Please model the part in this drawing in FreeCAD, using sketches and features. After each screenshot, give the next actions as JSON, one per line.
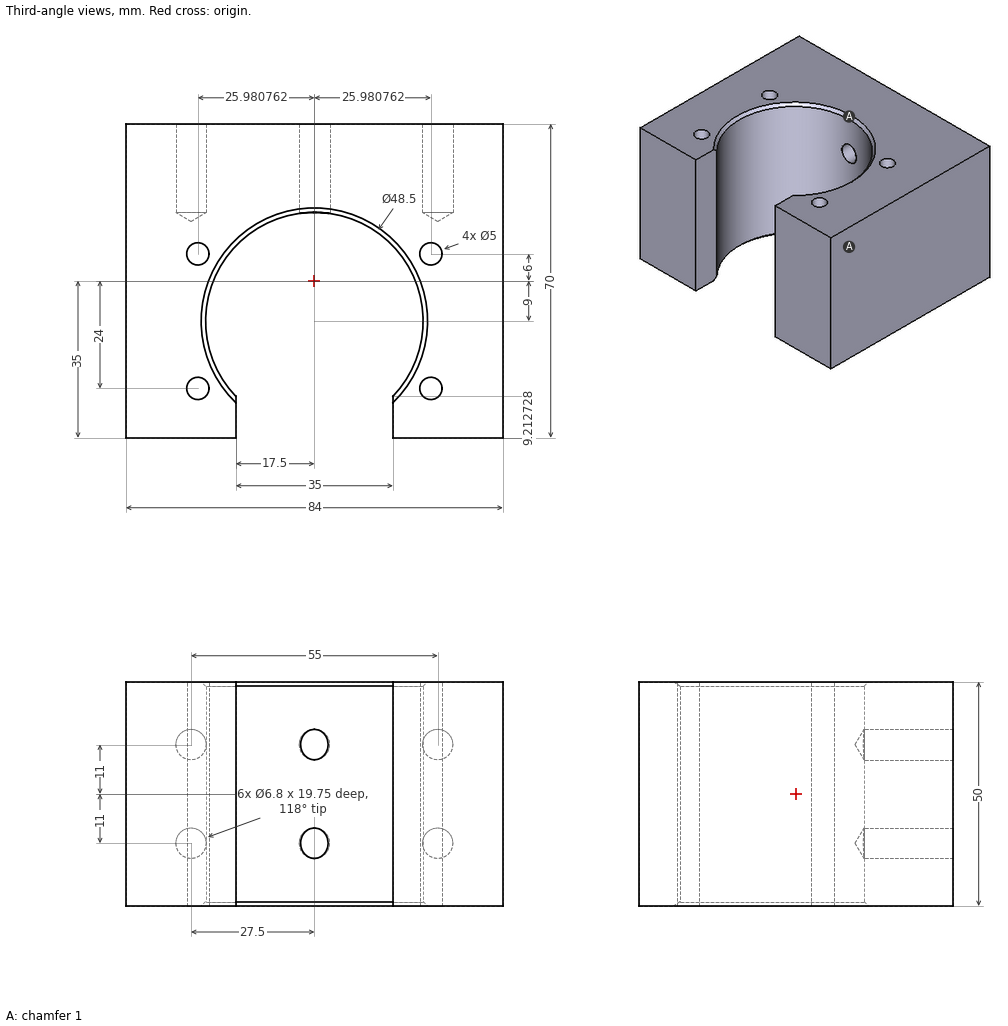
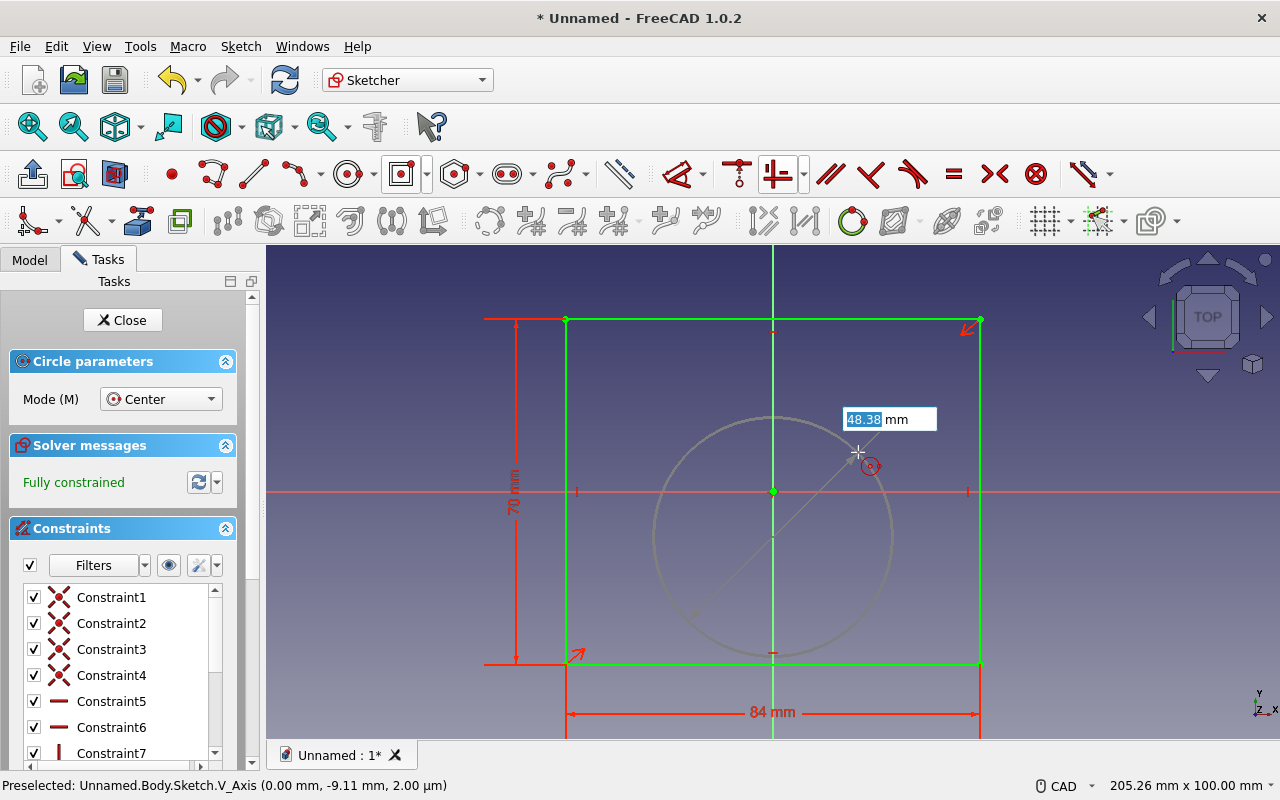
{"action": "type", "text": "48.5"}
{"action": "key", "text": "Return"}
{"action": "key", "text": "Escape"}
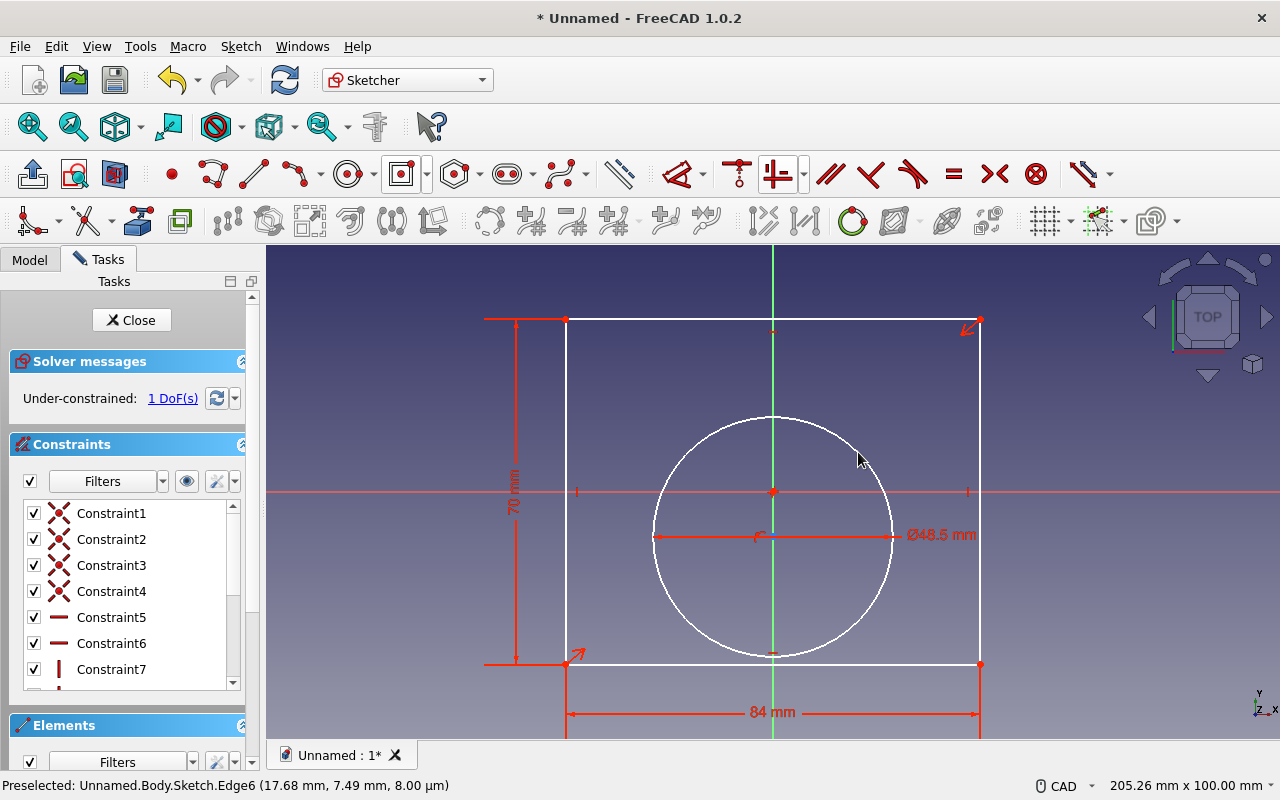
{"action": "key", "text": "d"}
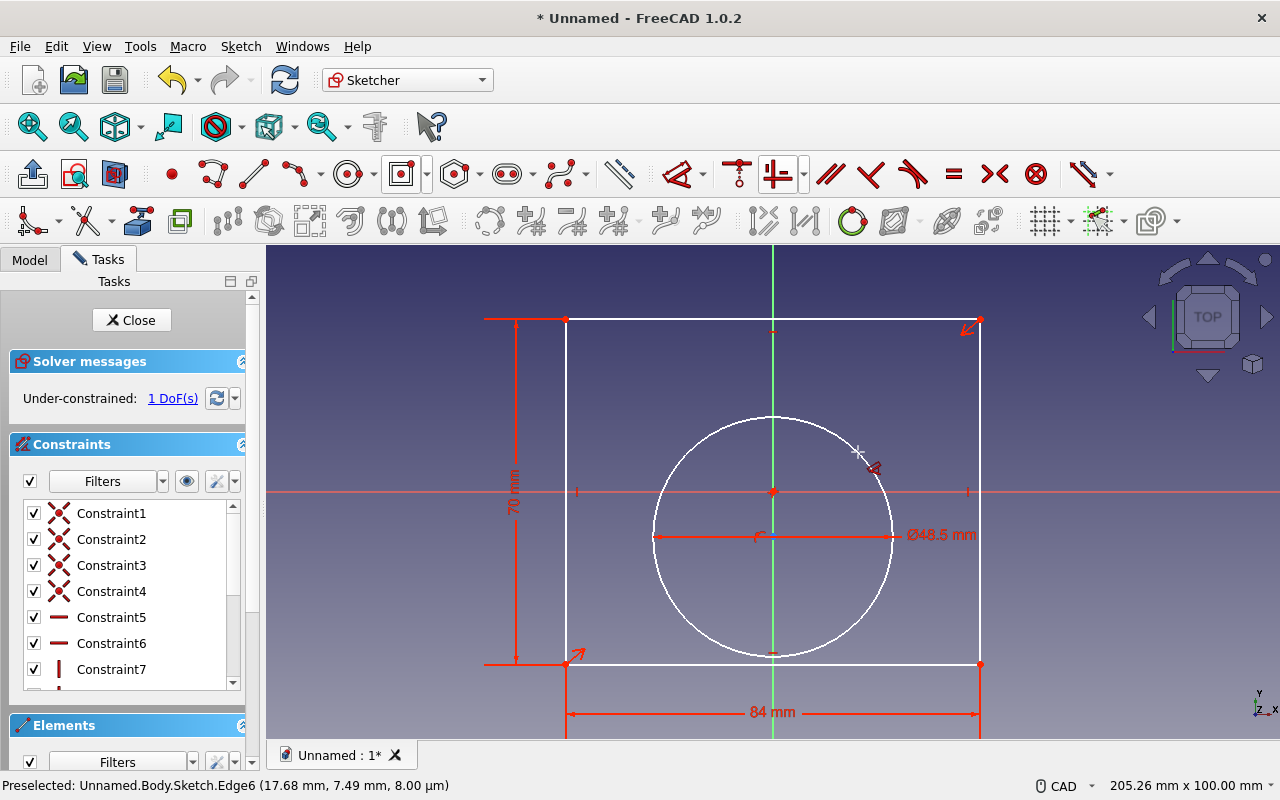
{"action": "left_click", "coordinate": [773, 537]}
{"action": "left_click", "coordinate": [807, 515]}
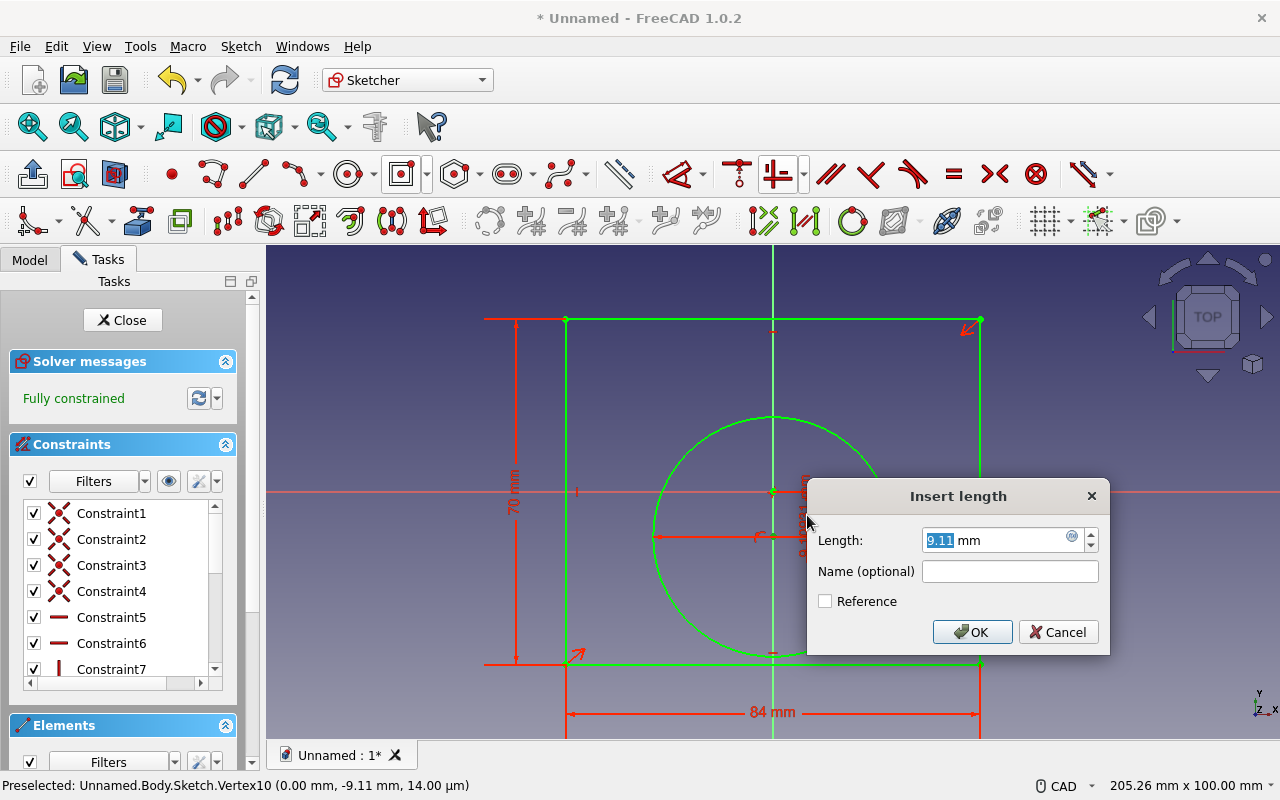
{"action": "type", "text": "9"}
{"action": "key", "text": "Return"}
{"action": "key", "text": "Escape"}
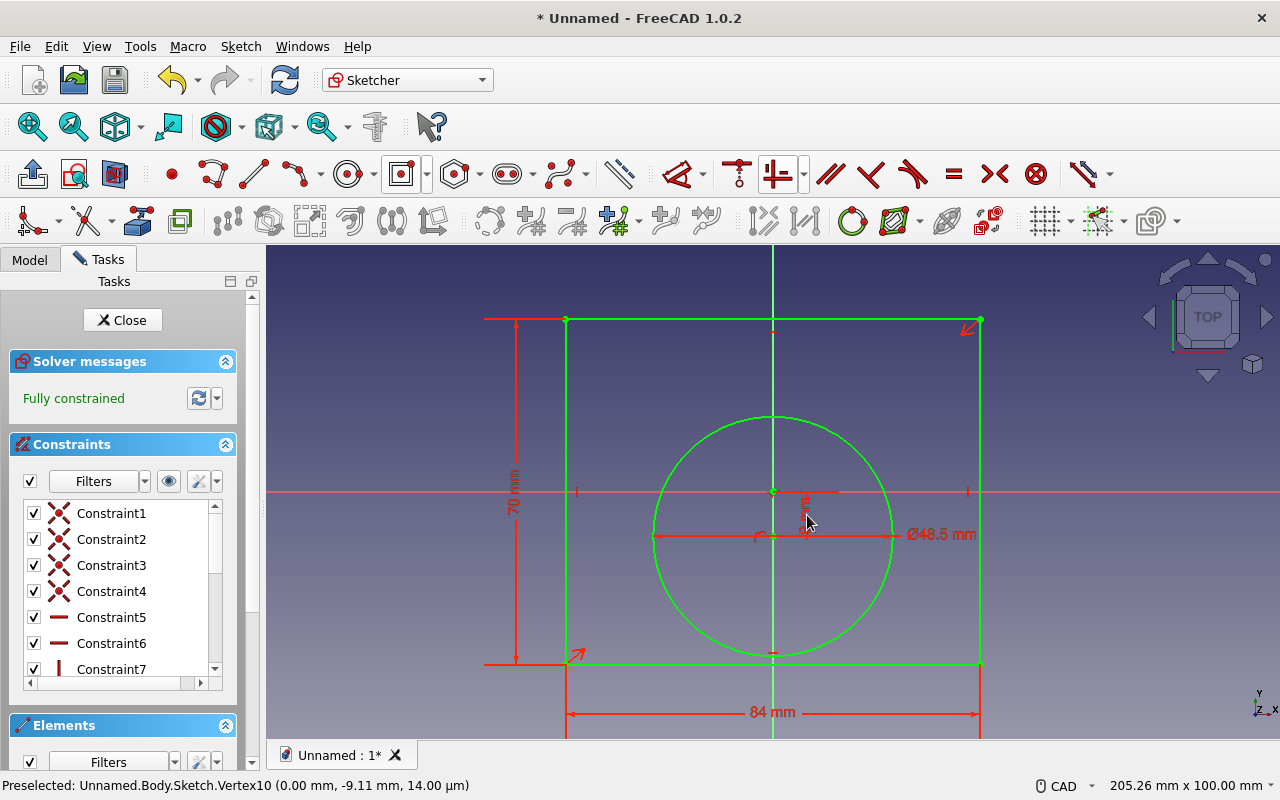
{"action": "left_click", "coordinate": [123, 320]}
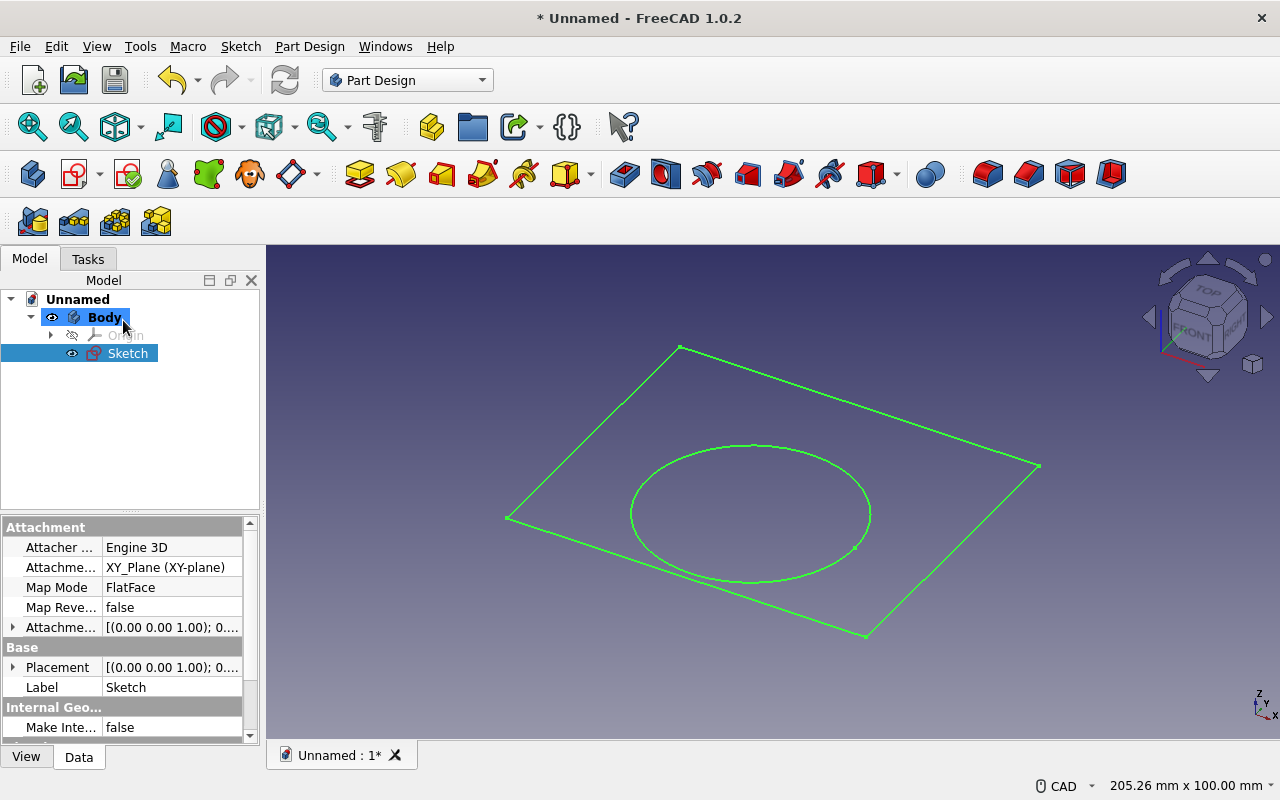
{"action": "left_click", "coordinate": [360, 174]}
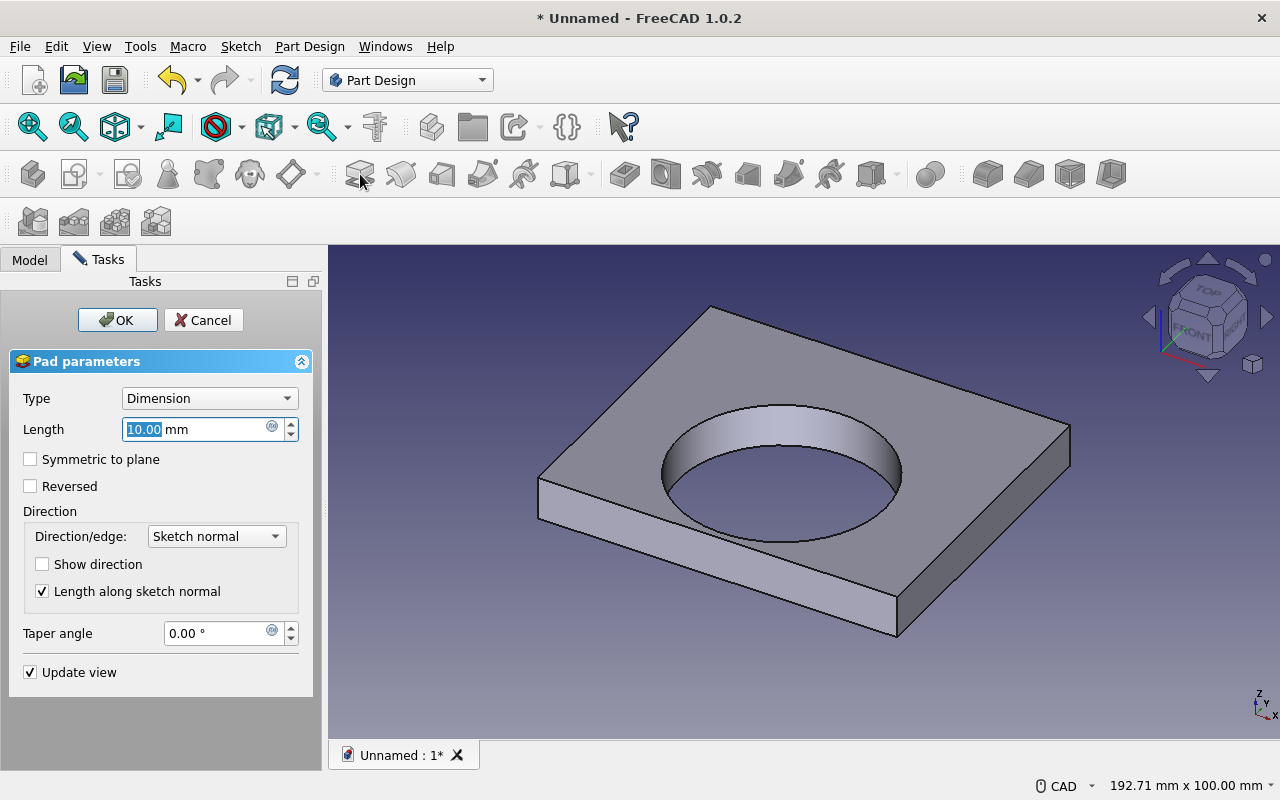
{"action": "type", "text": "50"}
{"action": "key", "text": "Tab"}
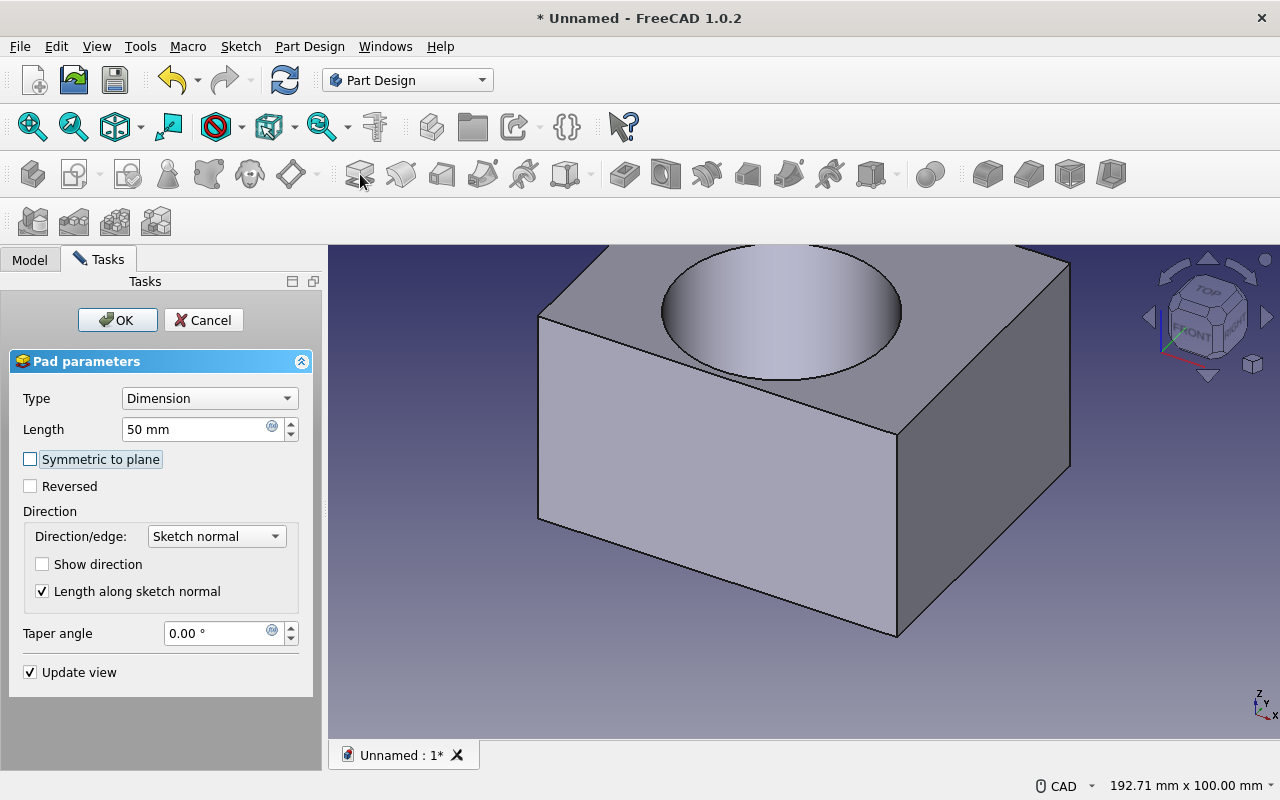
{"action": "left_click", "coordinate": [31, 459]}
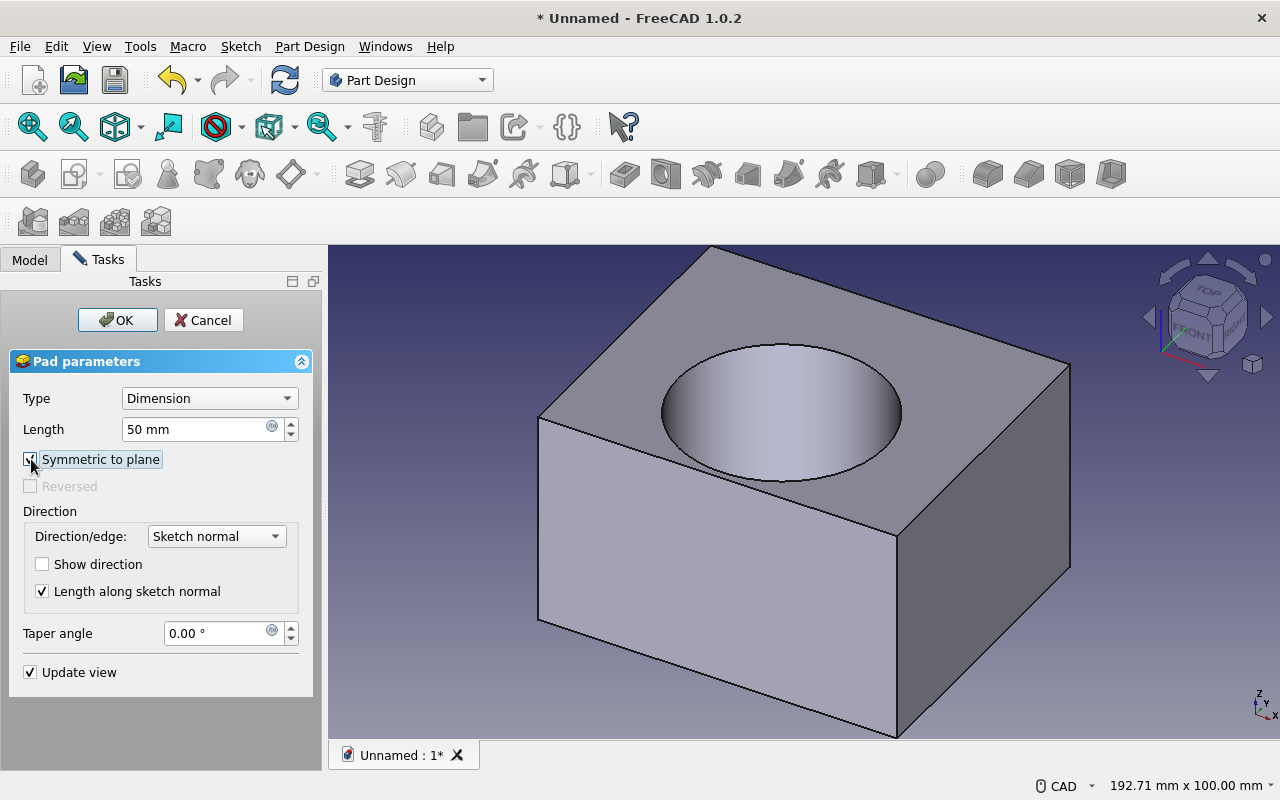
{"action": "left_click", "coordinate": [118, 320]}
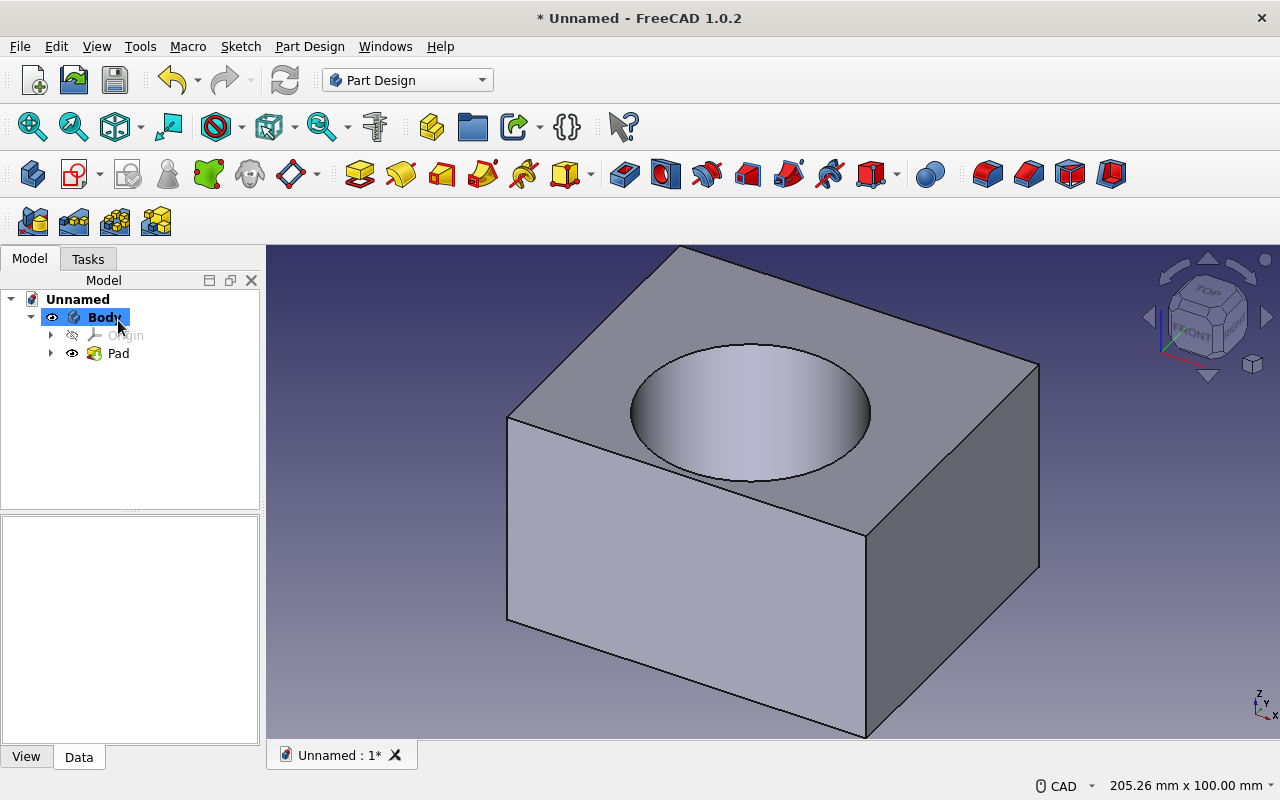
{"action": "left_click", "coordinate": [33, 128]}